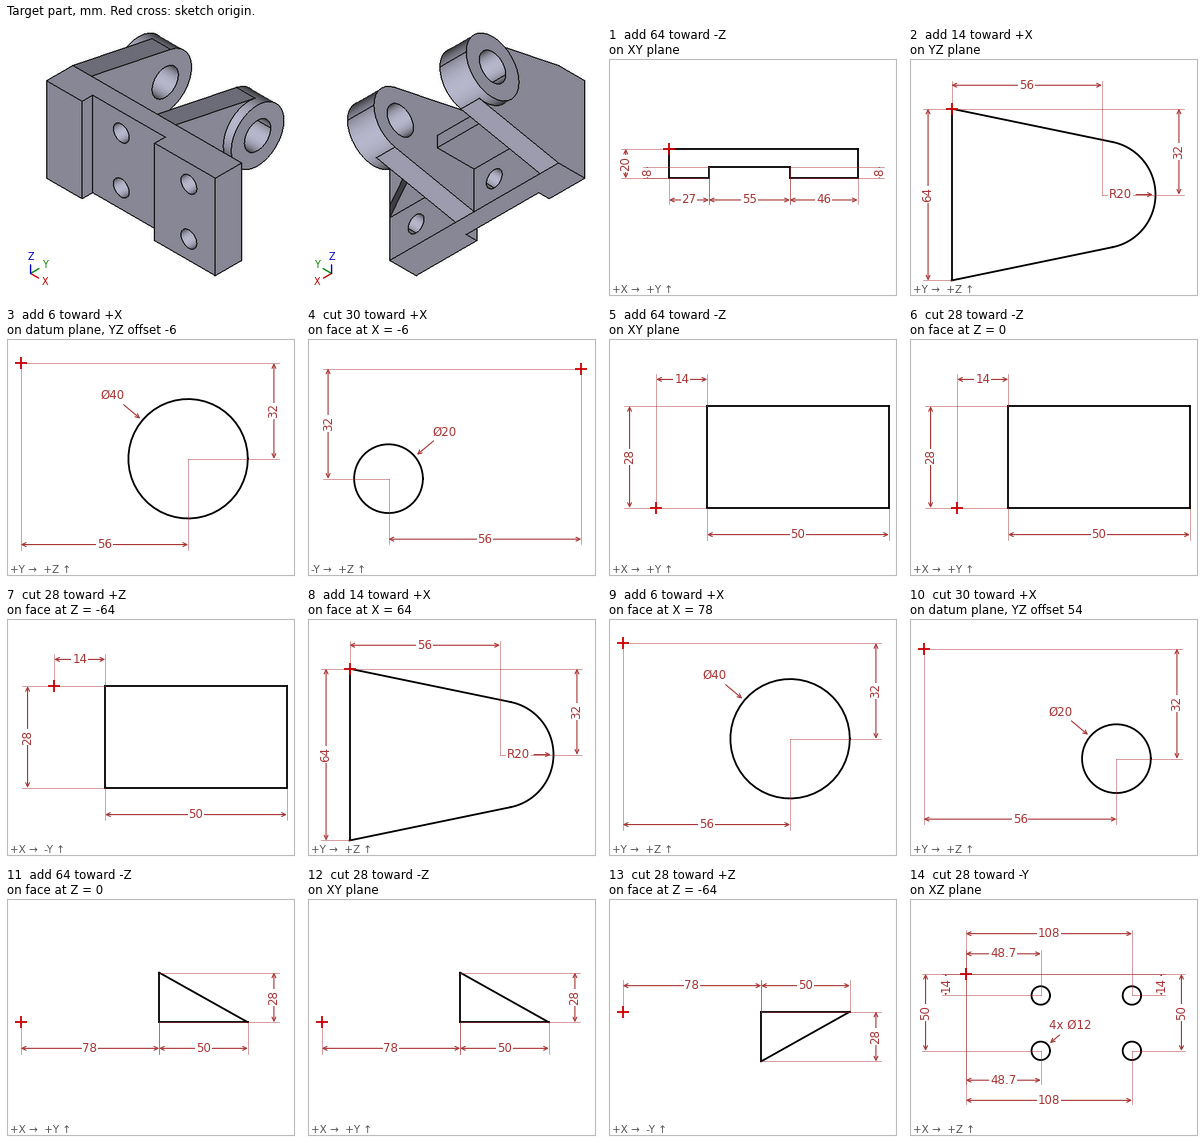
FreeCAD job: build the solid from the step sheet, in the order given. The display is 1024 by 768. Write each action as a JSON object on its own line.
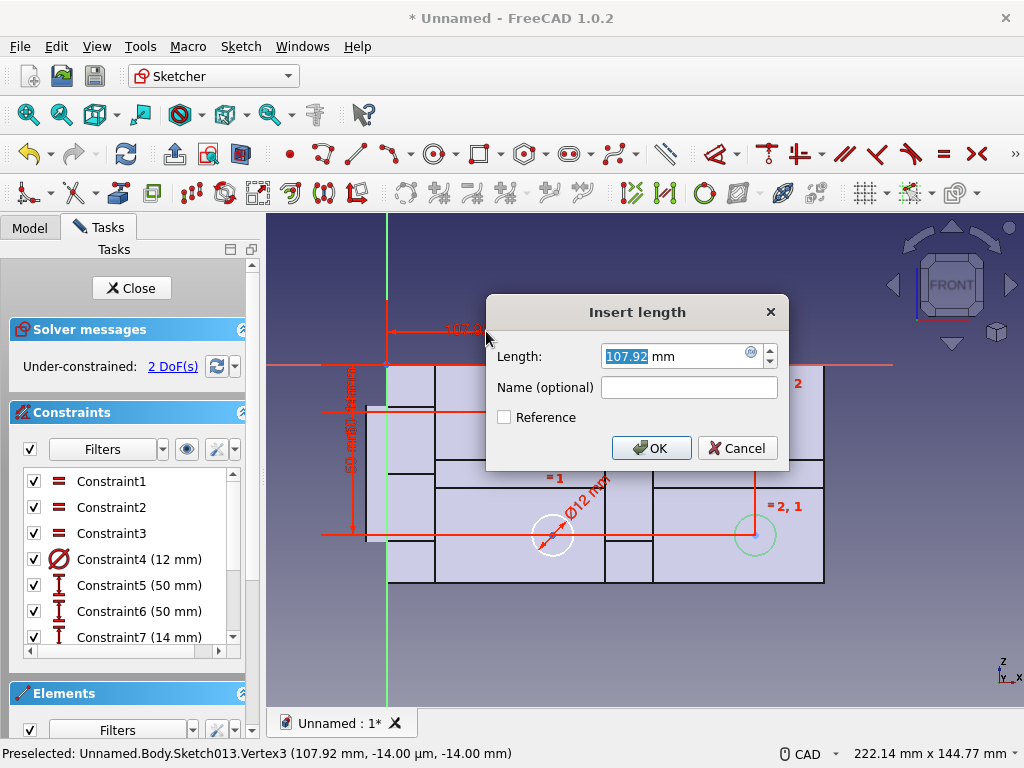
{"action": "type", "text": "108"}
{"action": "key", "text": "Return"}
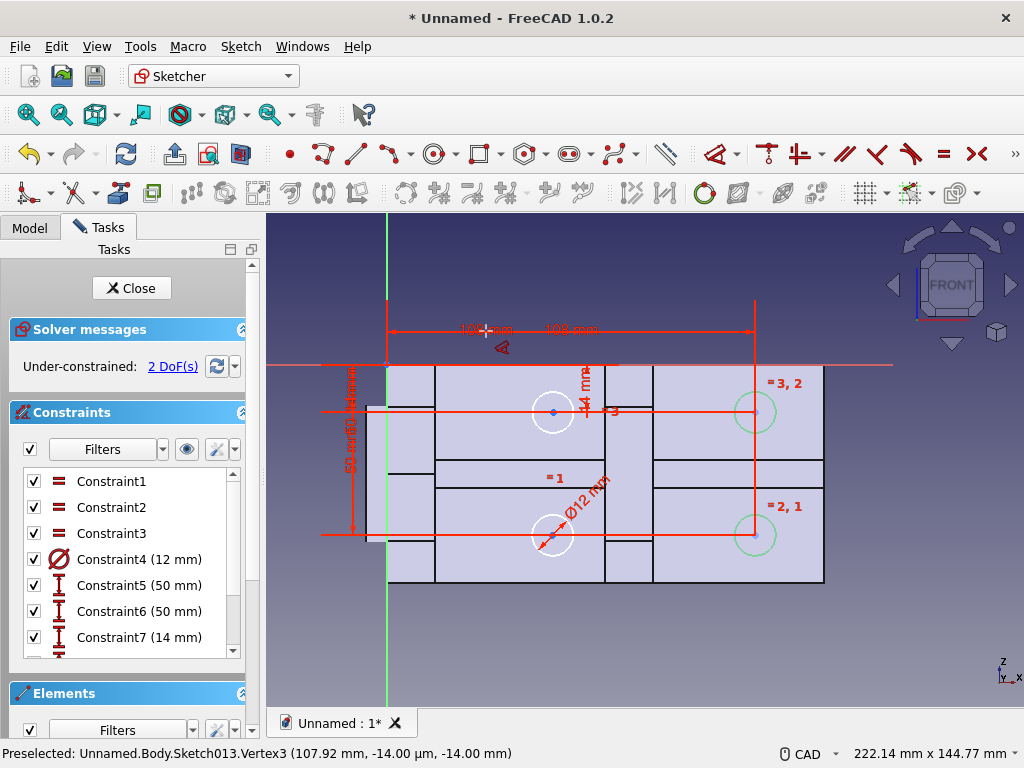
{"action": "left_click", "coordinate": [553, 535]}
{"action": "left_click", "coordinate": [412, 331]}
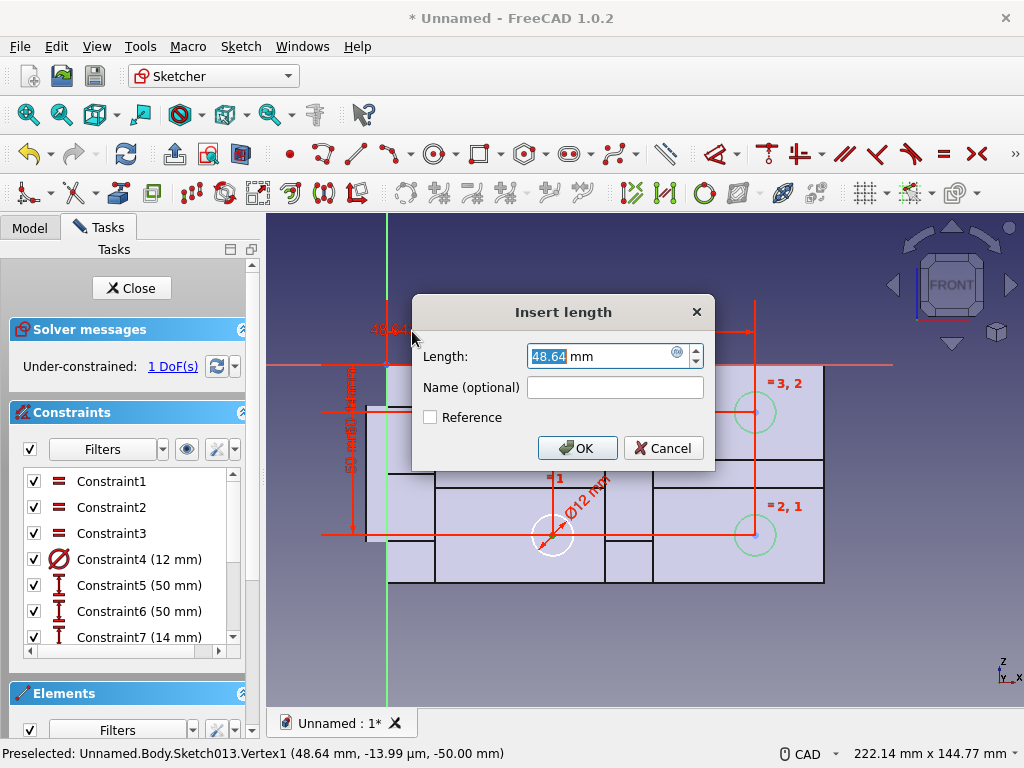
{"action": "type", "text": "48.7"}
{"action": "key", "text": "Return"}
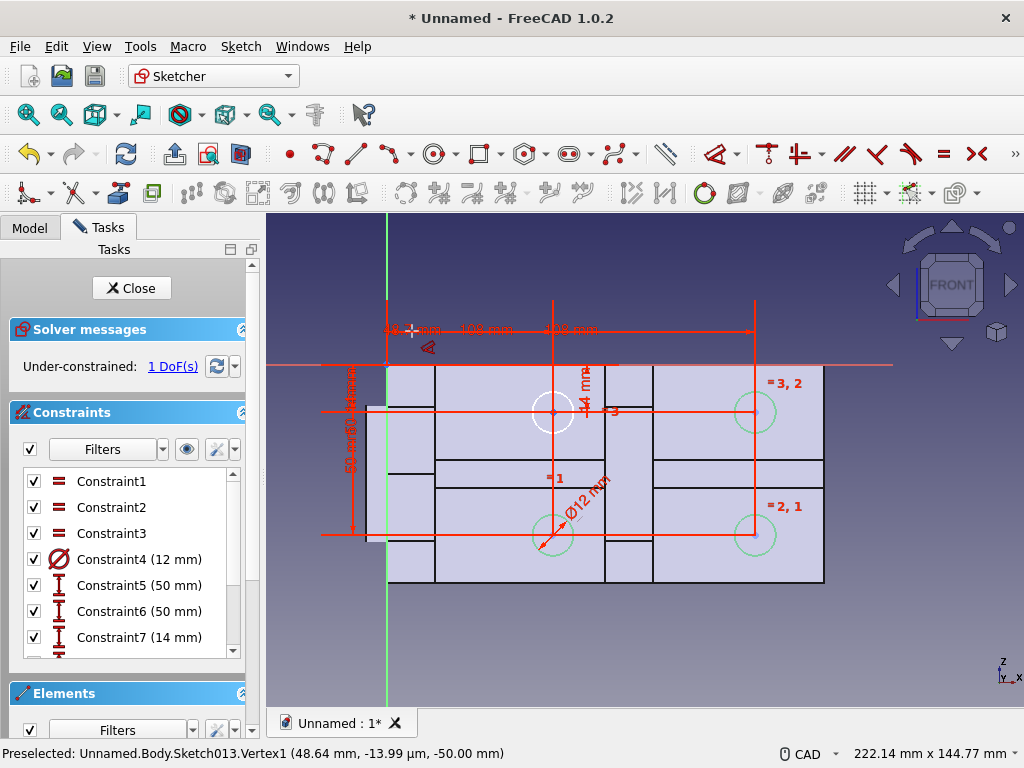
{"action": "left_click", "coordinate": [553, 412]}
{"action": "left_click", "coordinate": [470, 446]}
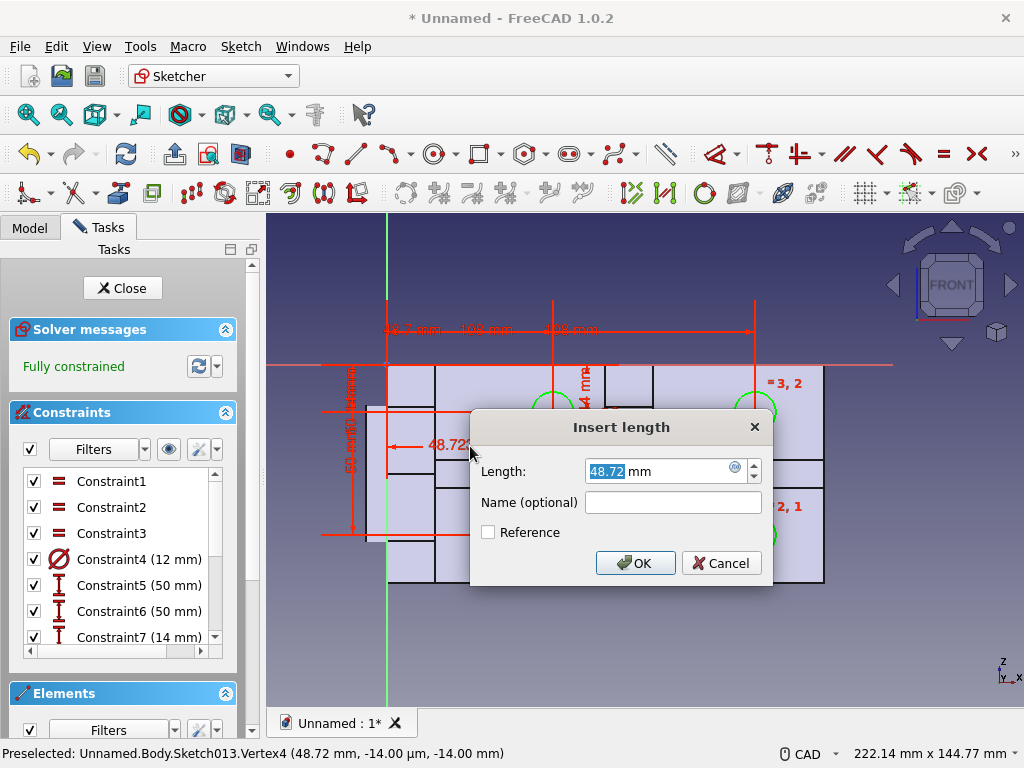
{"action": "type", "text": "48.7"}
{"action": "key", "text": "Return"}
{"action": "key", "text": "Escape"}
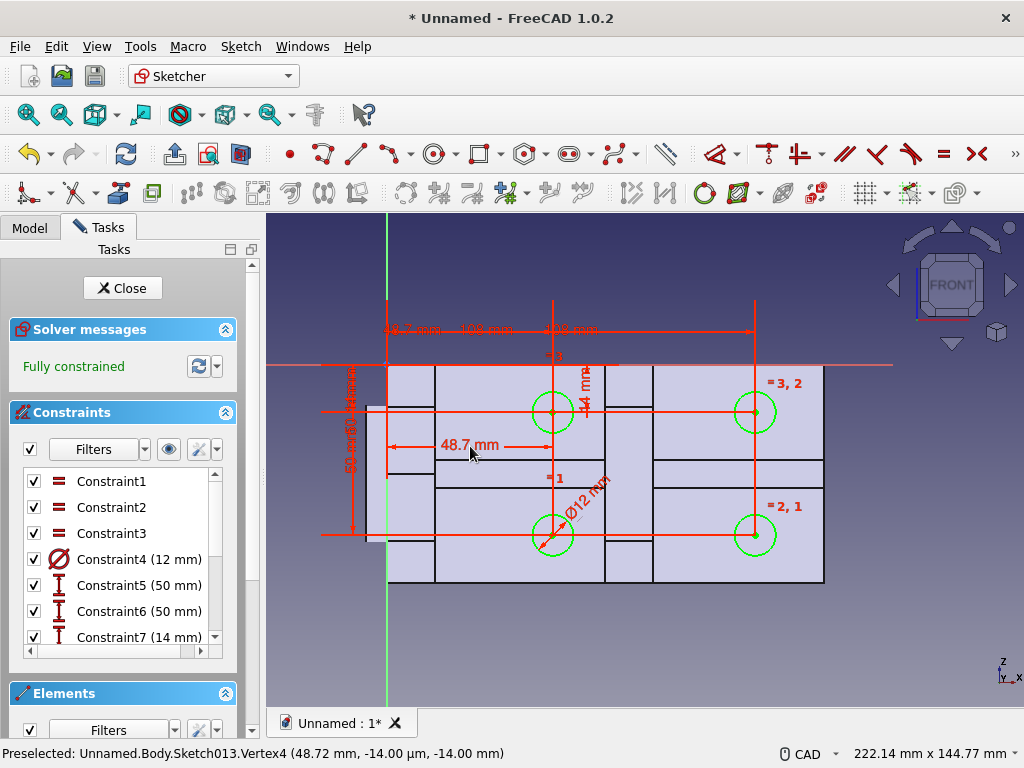
{"action": "left_click", "coordinate": [123, 288]}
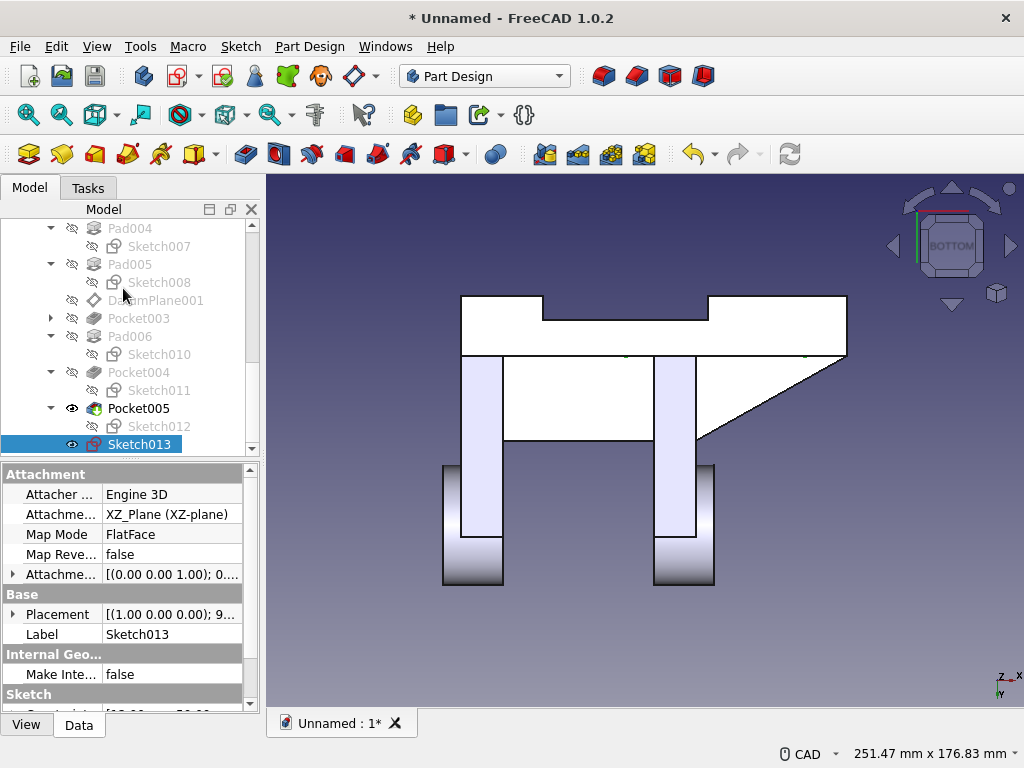
{"action": "left_click", "coordinate": [246, 154]}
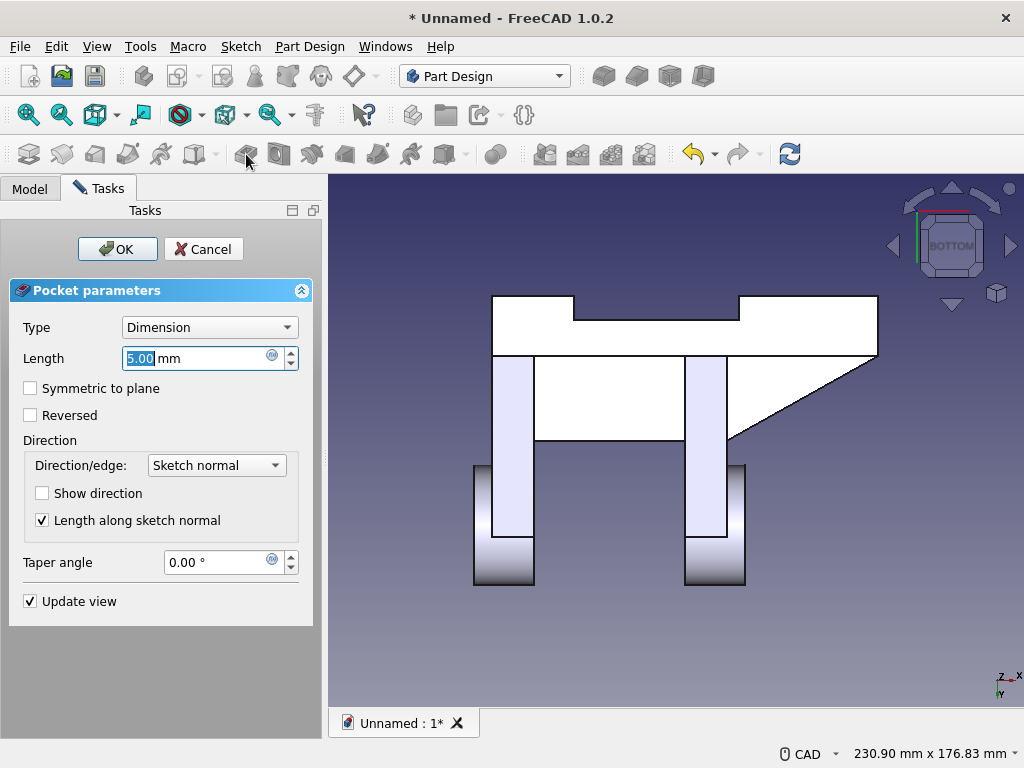
{"action": "type", "text": "28"}
{"action": "key", "text": "Tab"}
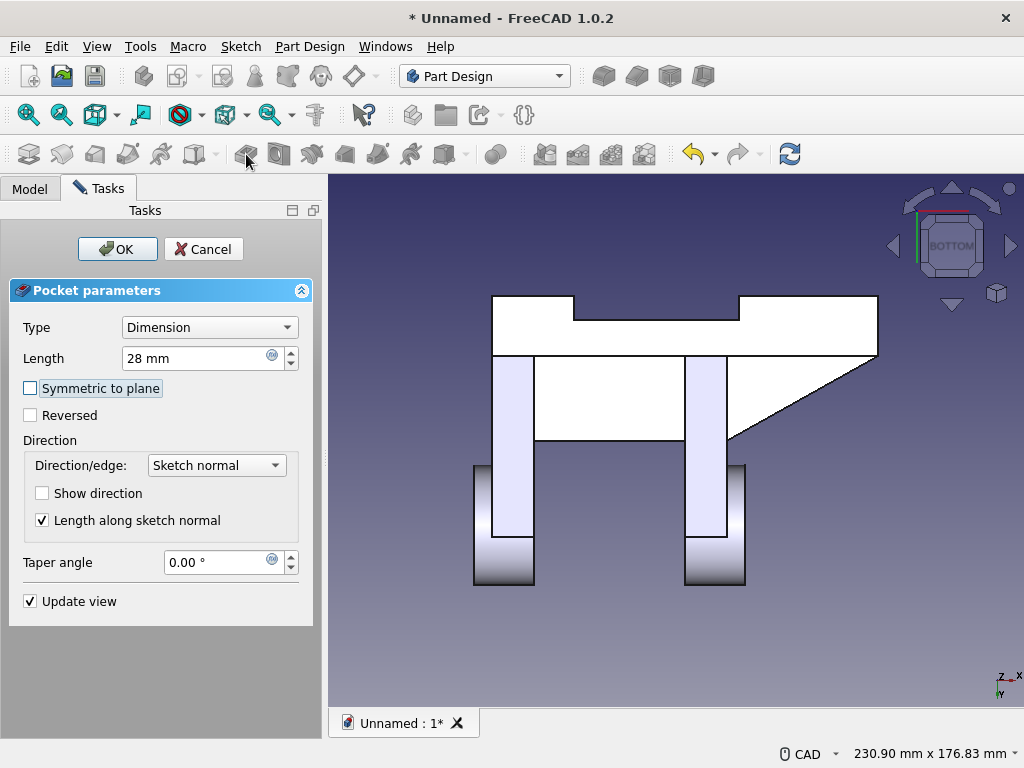
{"action": "left_click", "coordinate": [31, 415]}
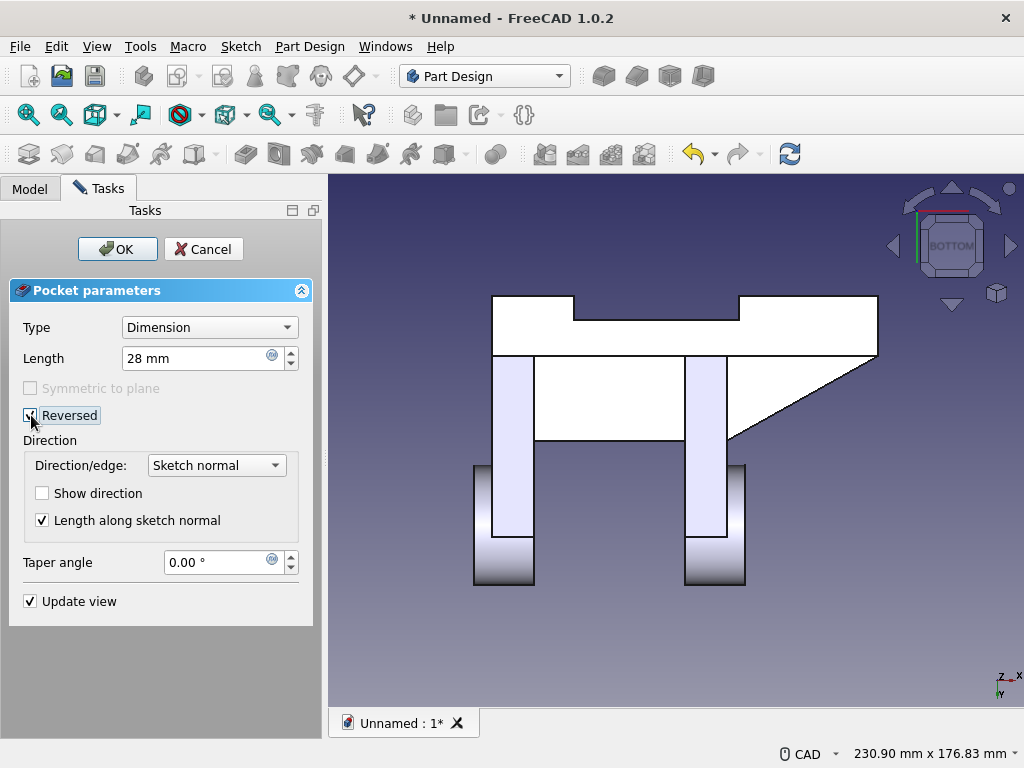
{"action": "left_click", "coordinate": [118, 249]}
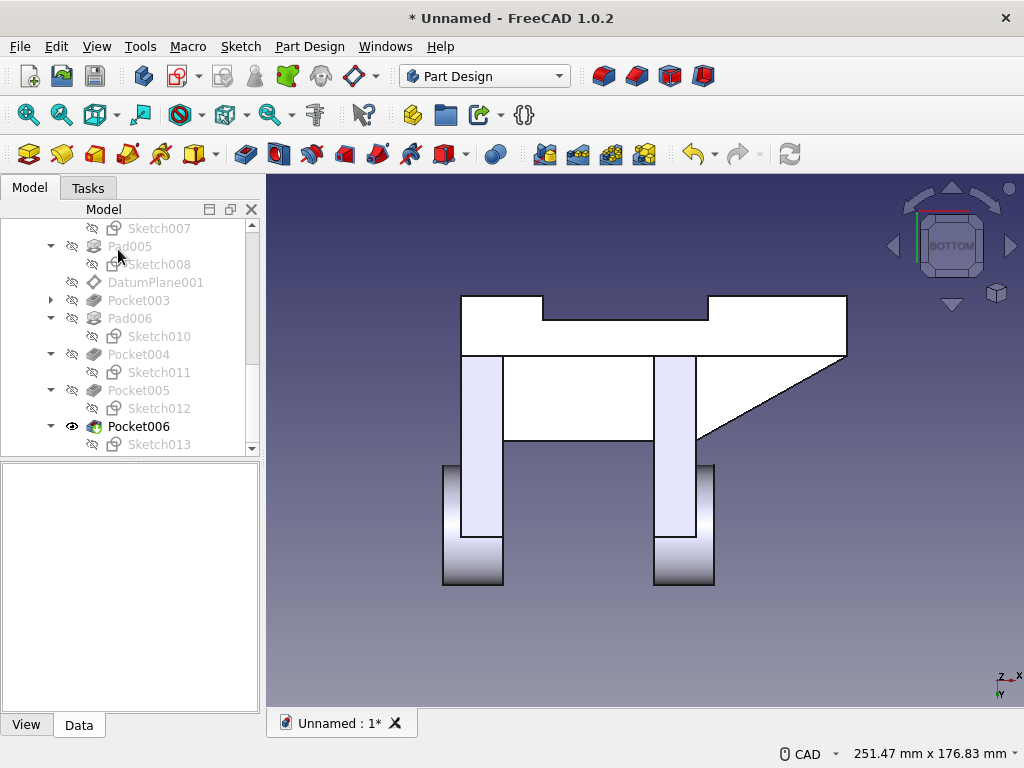
{"action": "key", "text": "0"}